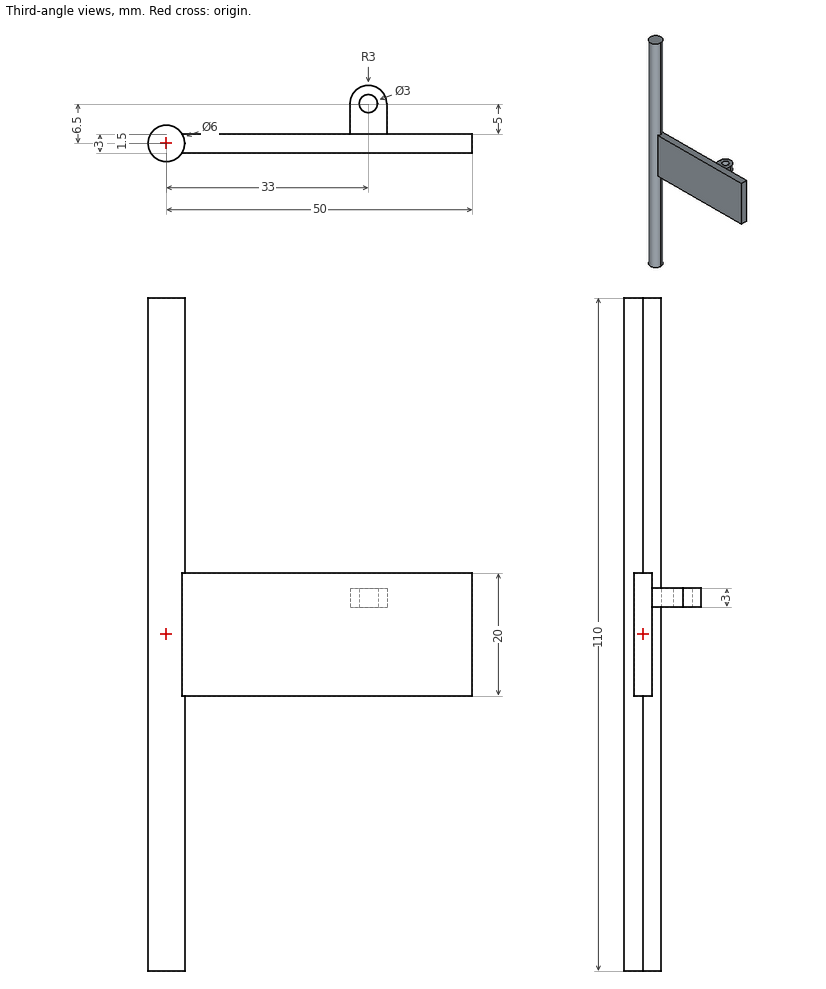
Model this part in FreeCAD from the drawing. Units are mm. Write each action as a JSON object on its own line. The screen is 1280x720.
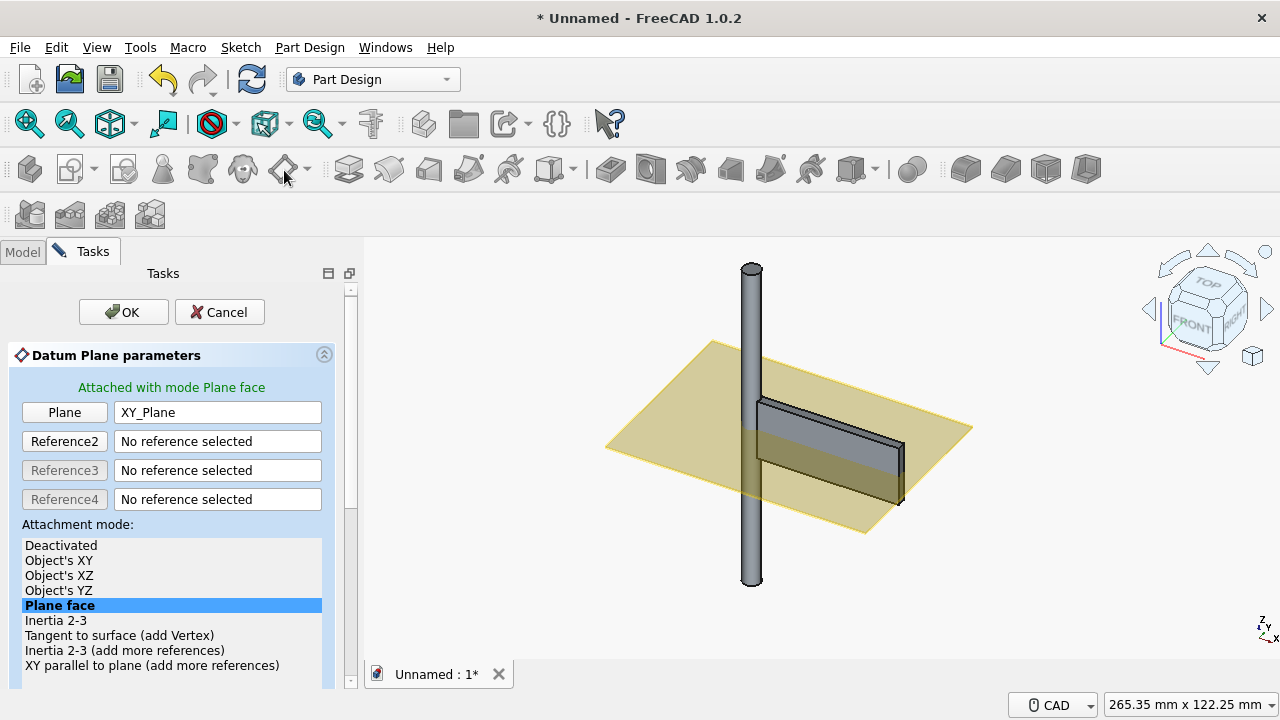
{"action": "scroll", "coordinate": [351, 486], "scroll_direction": "down", "scroll_amount": 4}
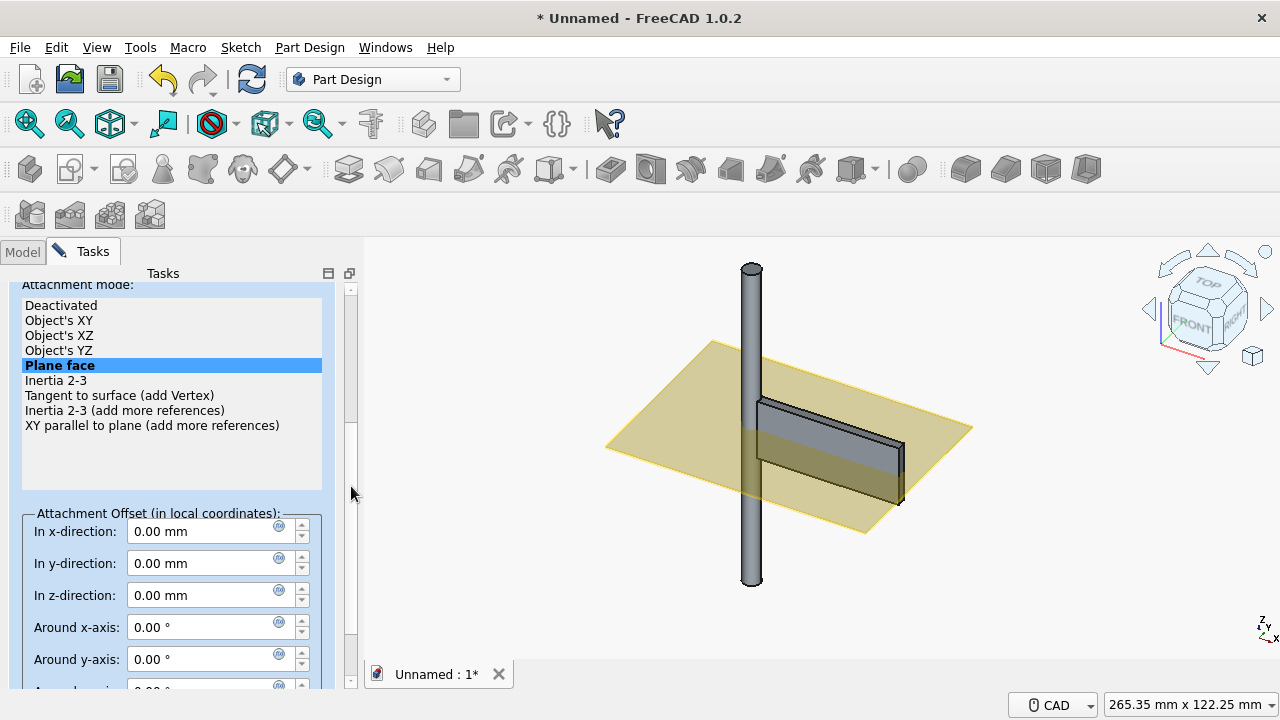
{"action": "triple_click", "coordinate": [210, 595]}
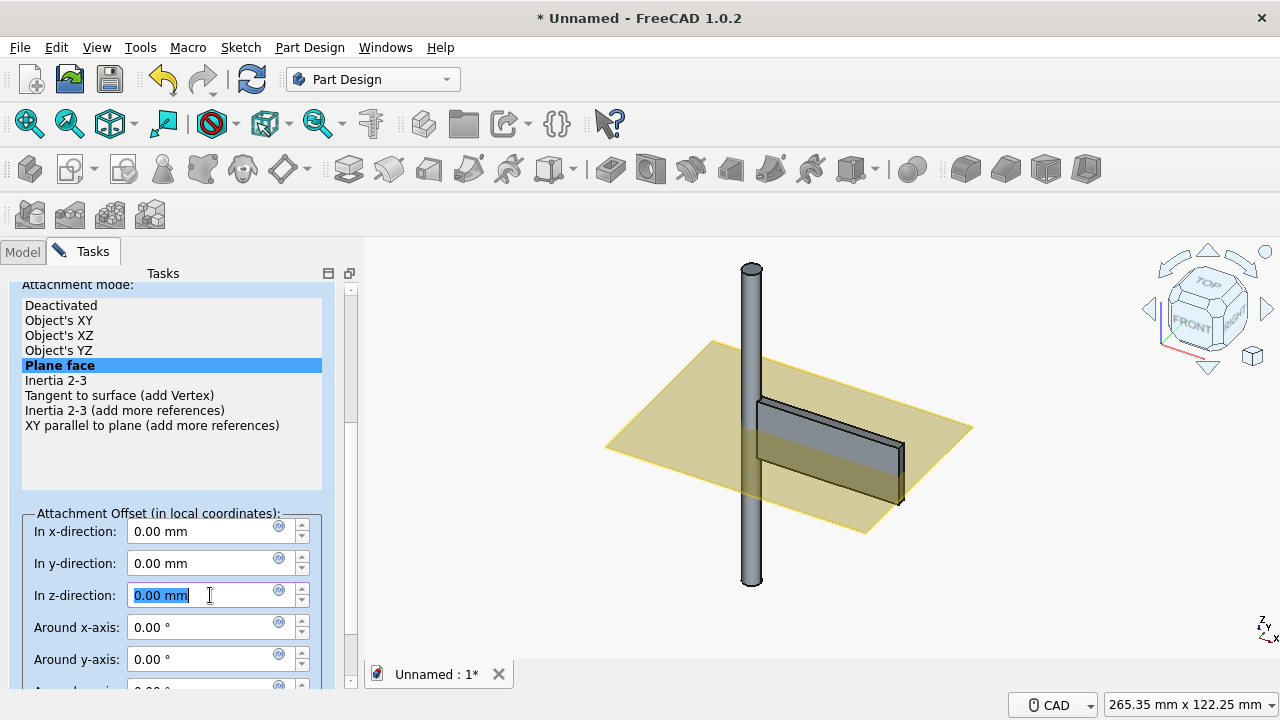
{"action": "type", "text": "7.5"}
{"action": "key", "text": "Tab"}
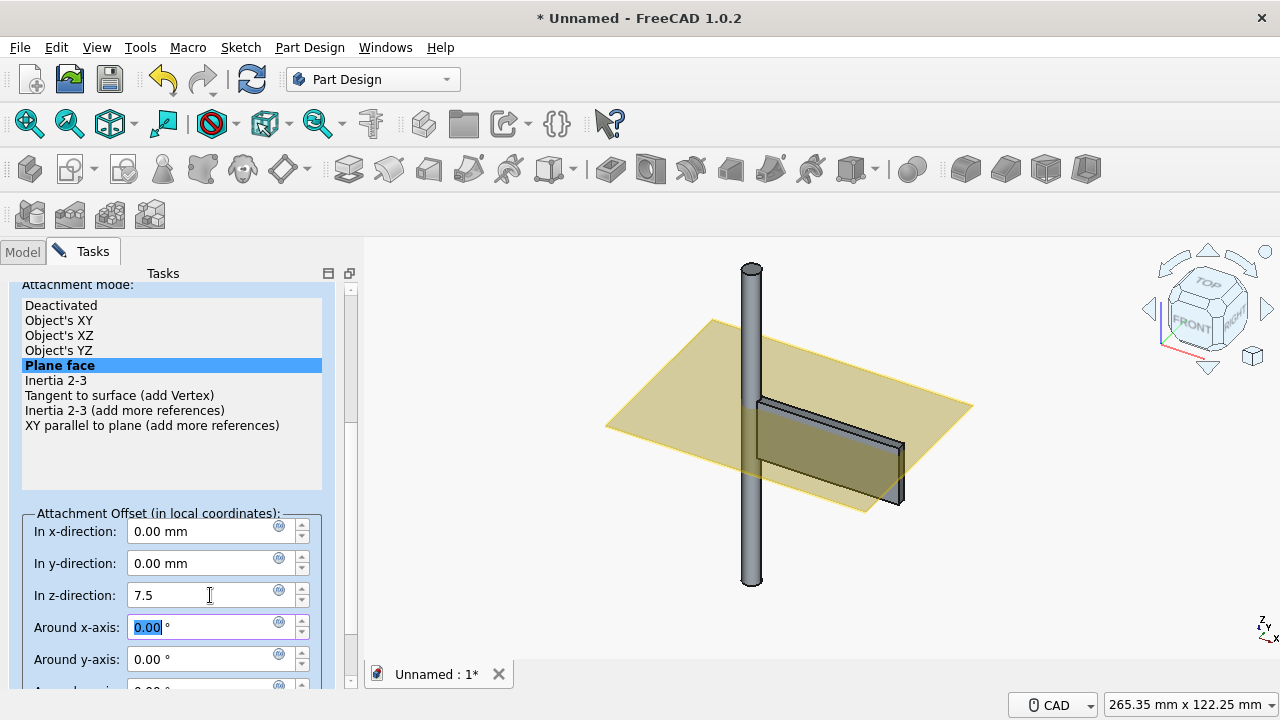
{"action": "scroll", "coordinate": [351, 486], "scroll_direction": "up", "scroll_amount": 5}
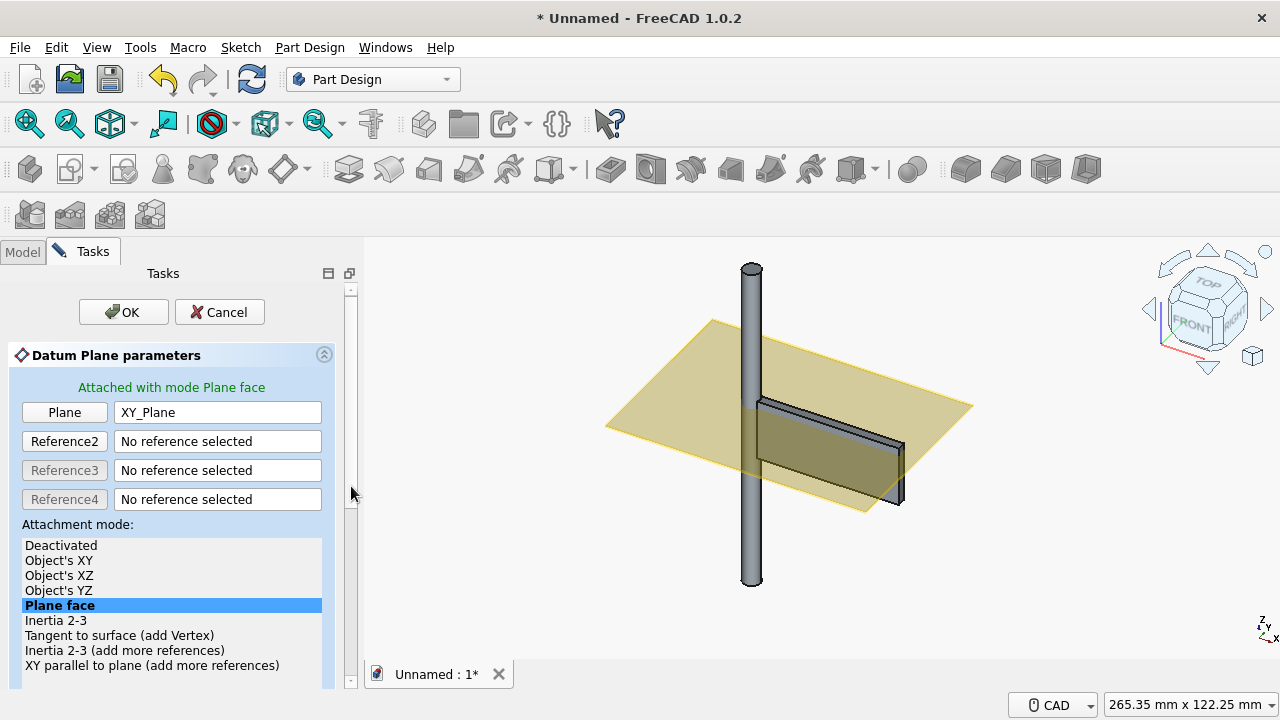
{"action": "left_click", "coordinate": [124, 312]}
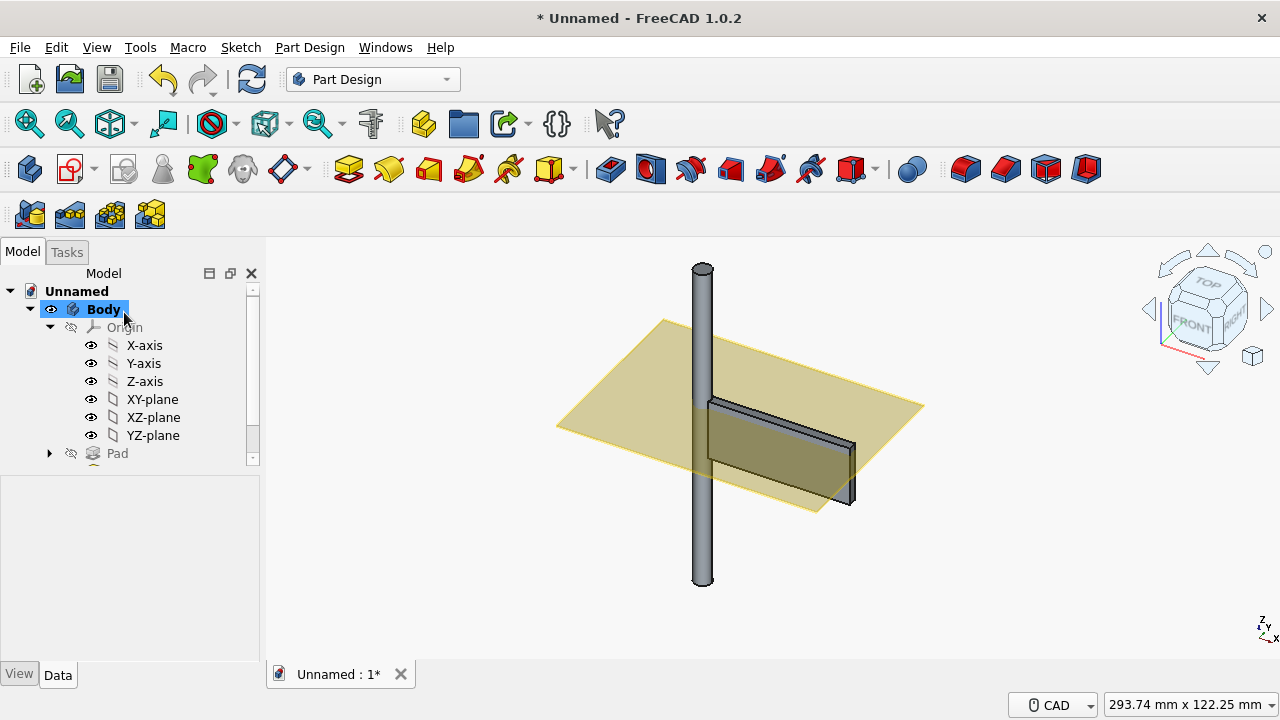
{"action": "scroll", "coordinate": [100, 377], "scroll_direction": "down", "scroll_amount": 3}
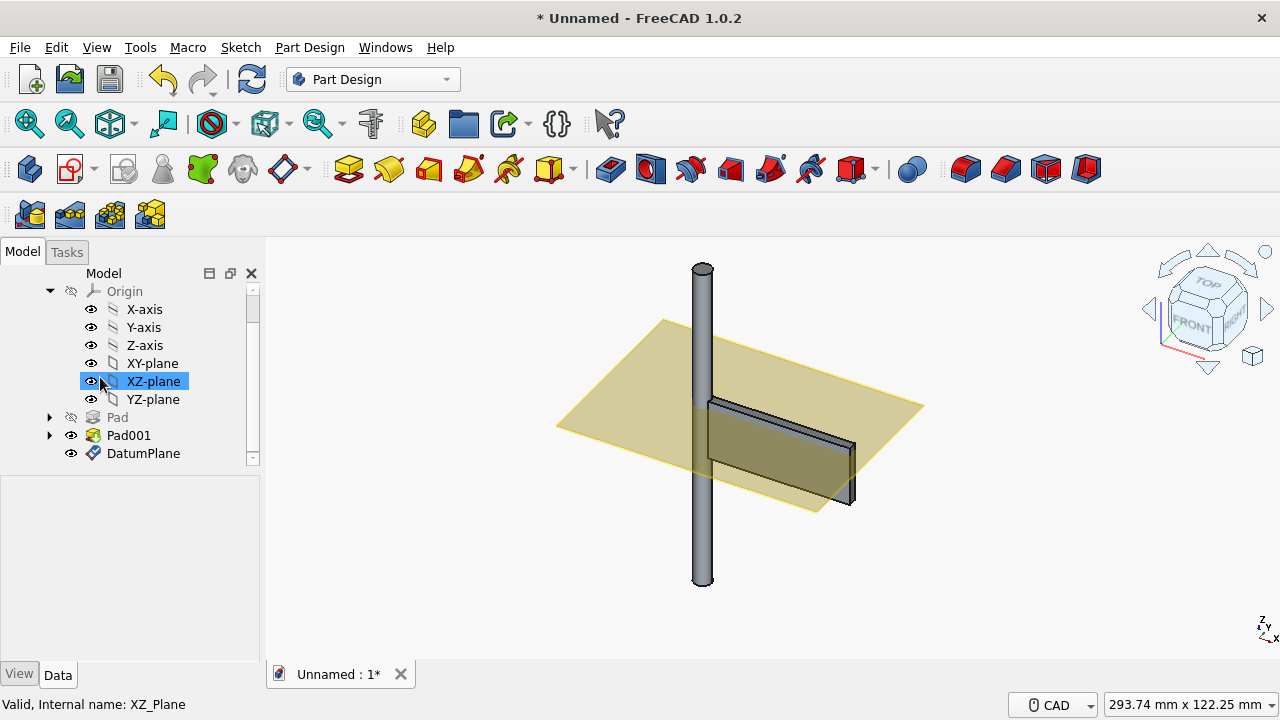
{"action": "left_click", "coordinate": [116, 453]}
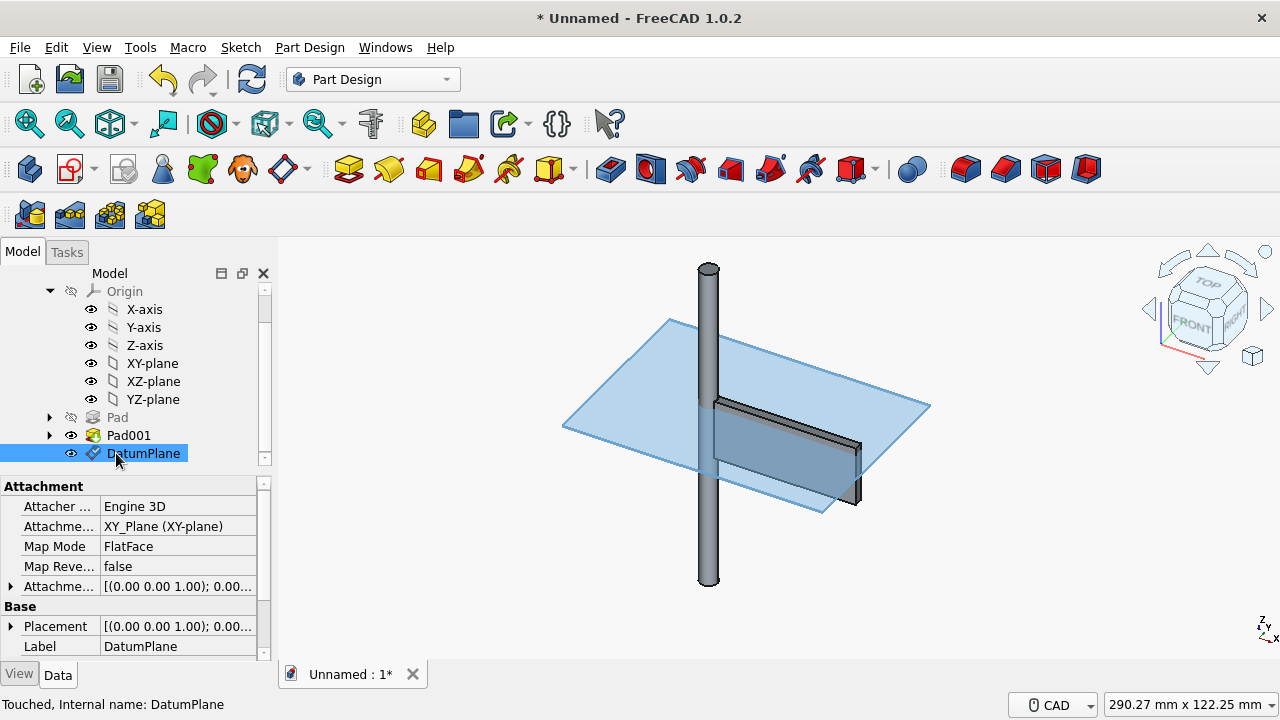
{"action": "left_click", "coordinate": [70, 170]}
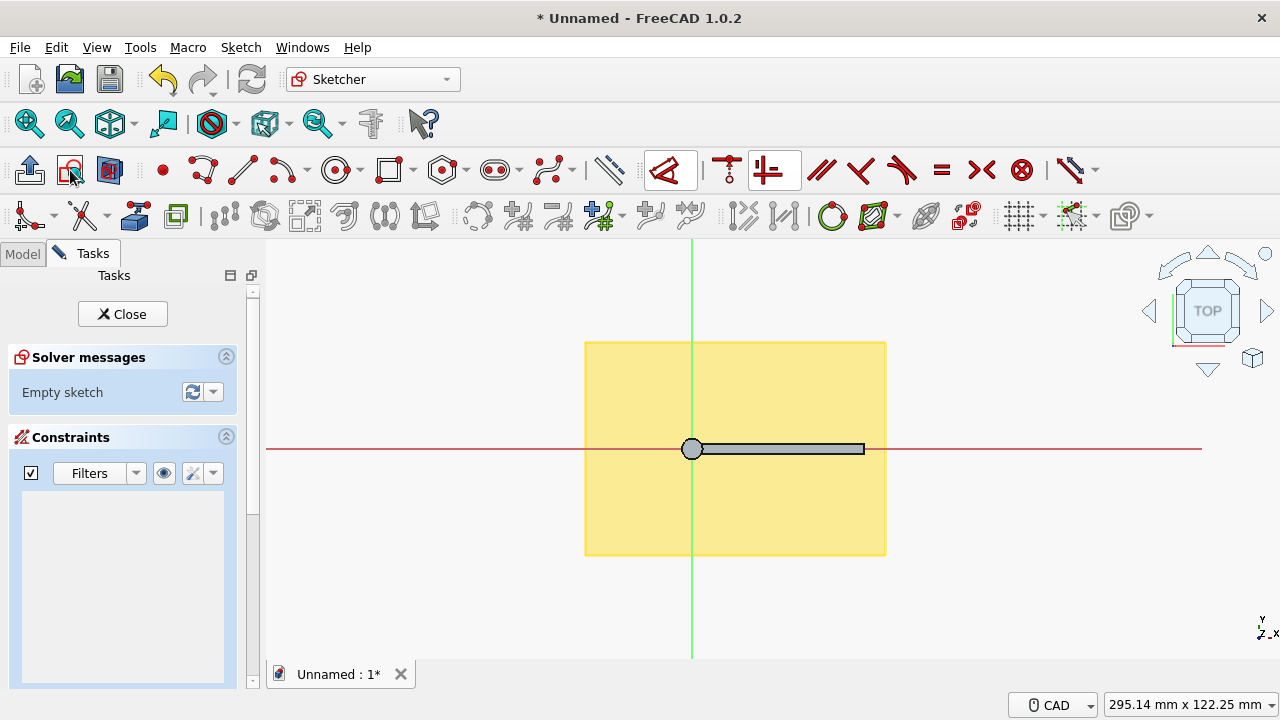
{"action": "left_click", "coordinate": [110, 170]}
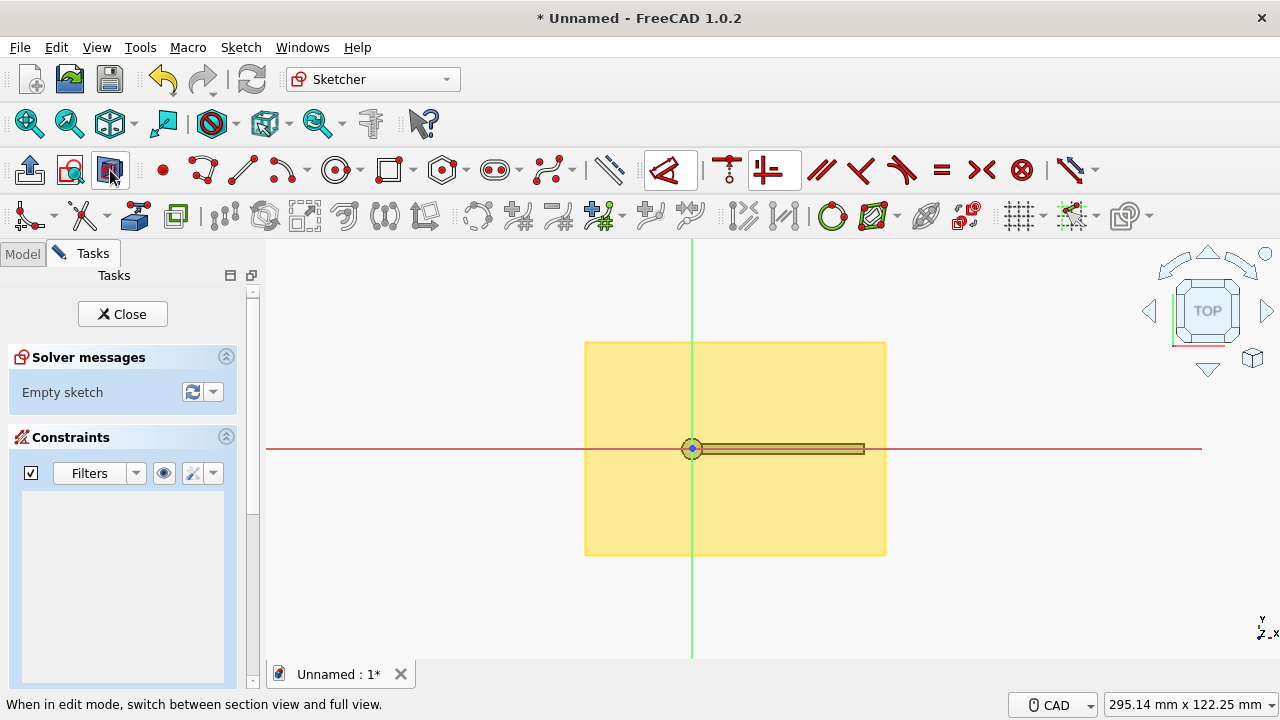
{"action": "scroll", "coordinate": [818, 428], "scroll_direction": "up", "scroll_amount": 11}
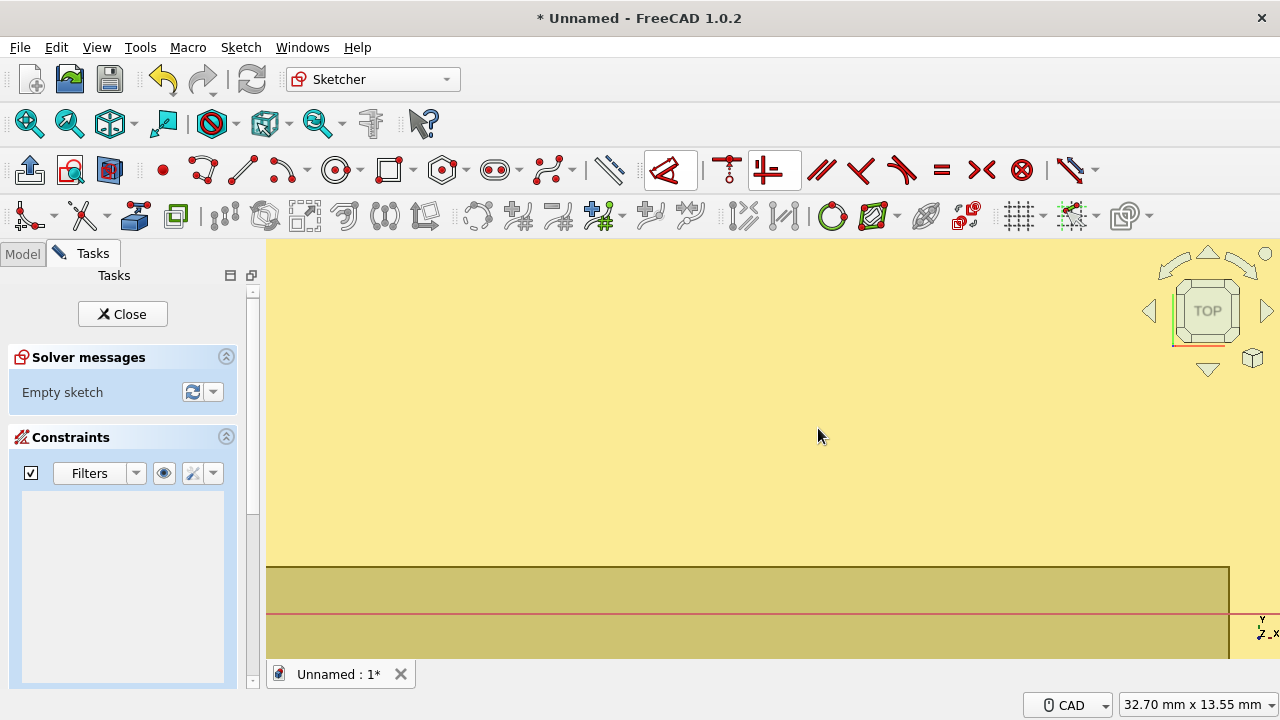
{"action": "left_click", "coordinate": [204, 170]}